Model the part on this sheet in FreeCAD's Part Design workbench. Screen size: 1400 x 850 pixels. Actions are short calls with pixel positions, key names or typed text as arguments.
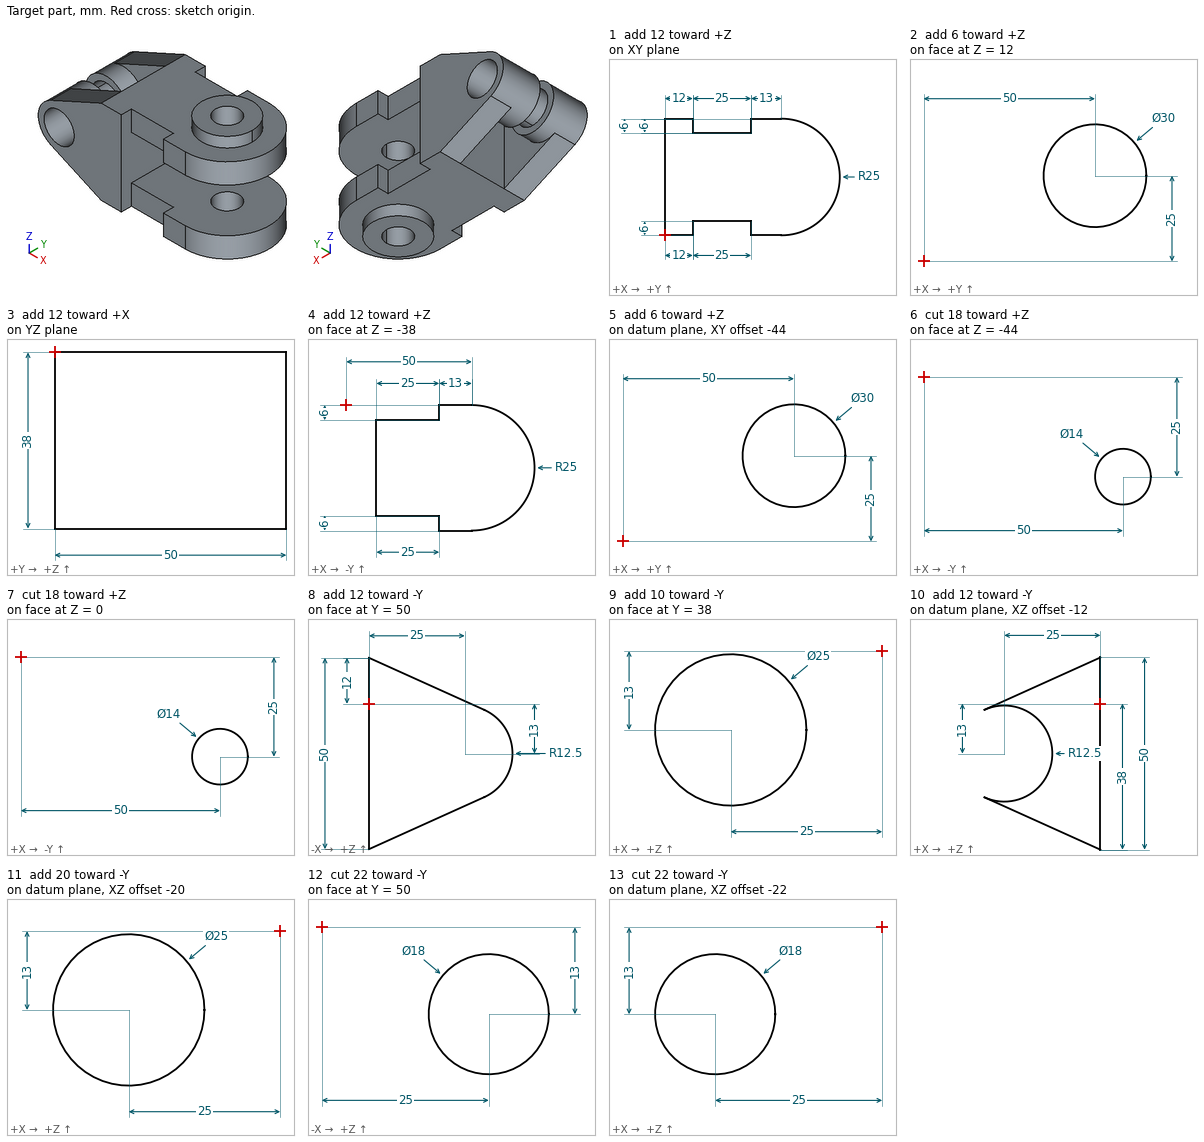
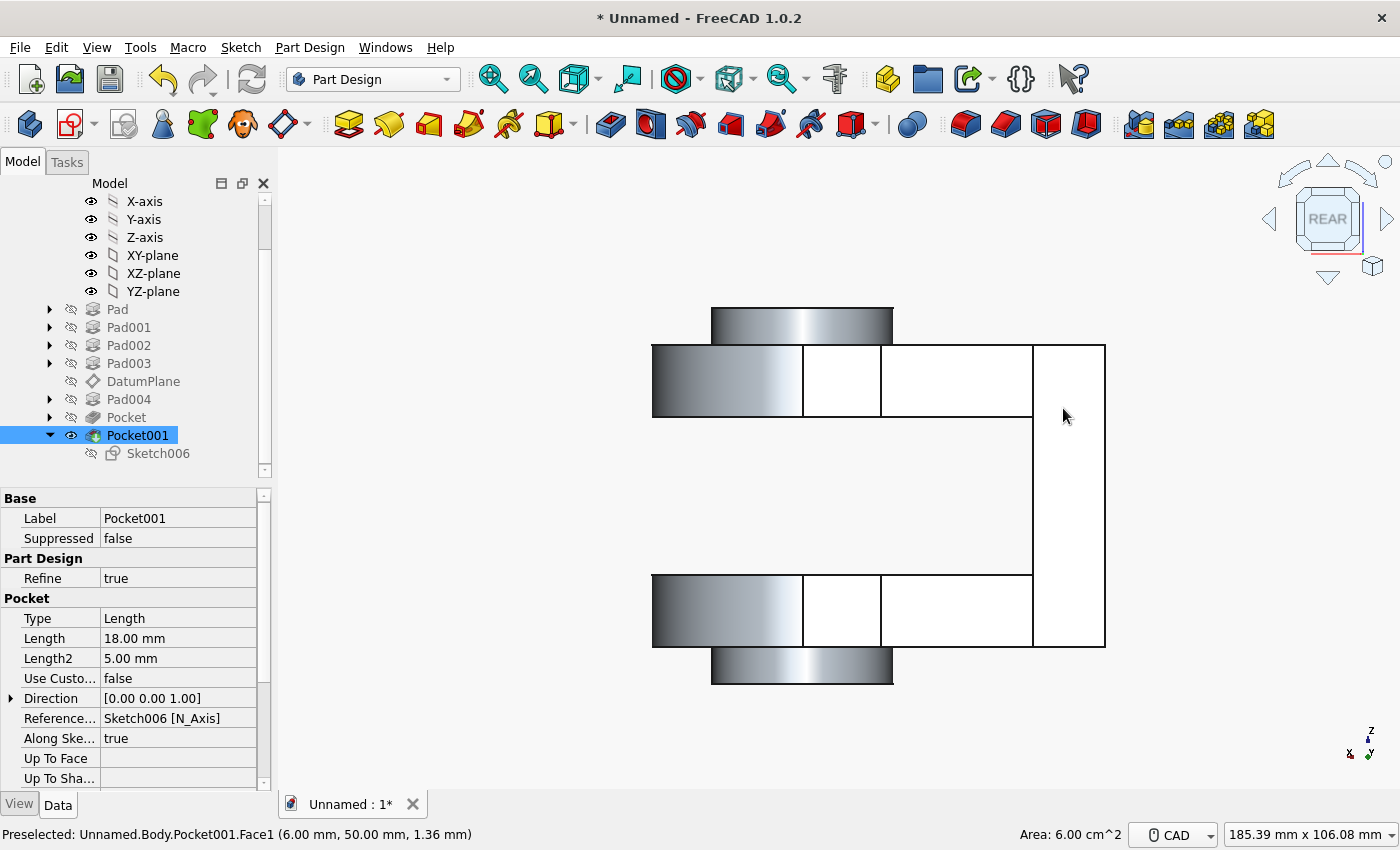
click(70, 124)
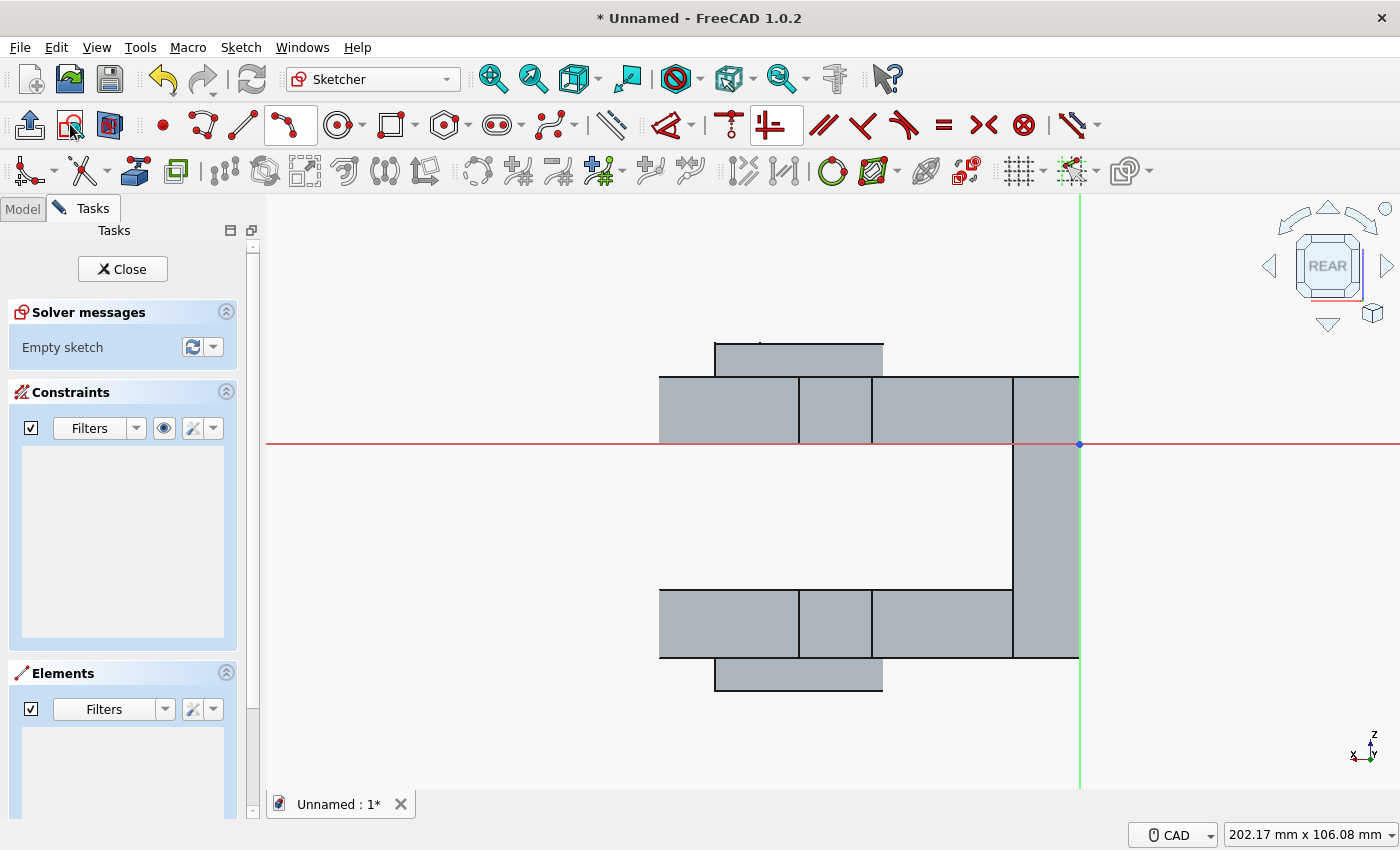
scroll(294, 375, down, 1)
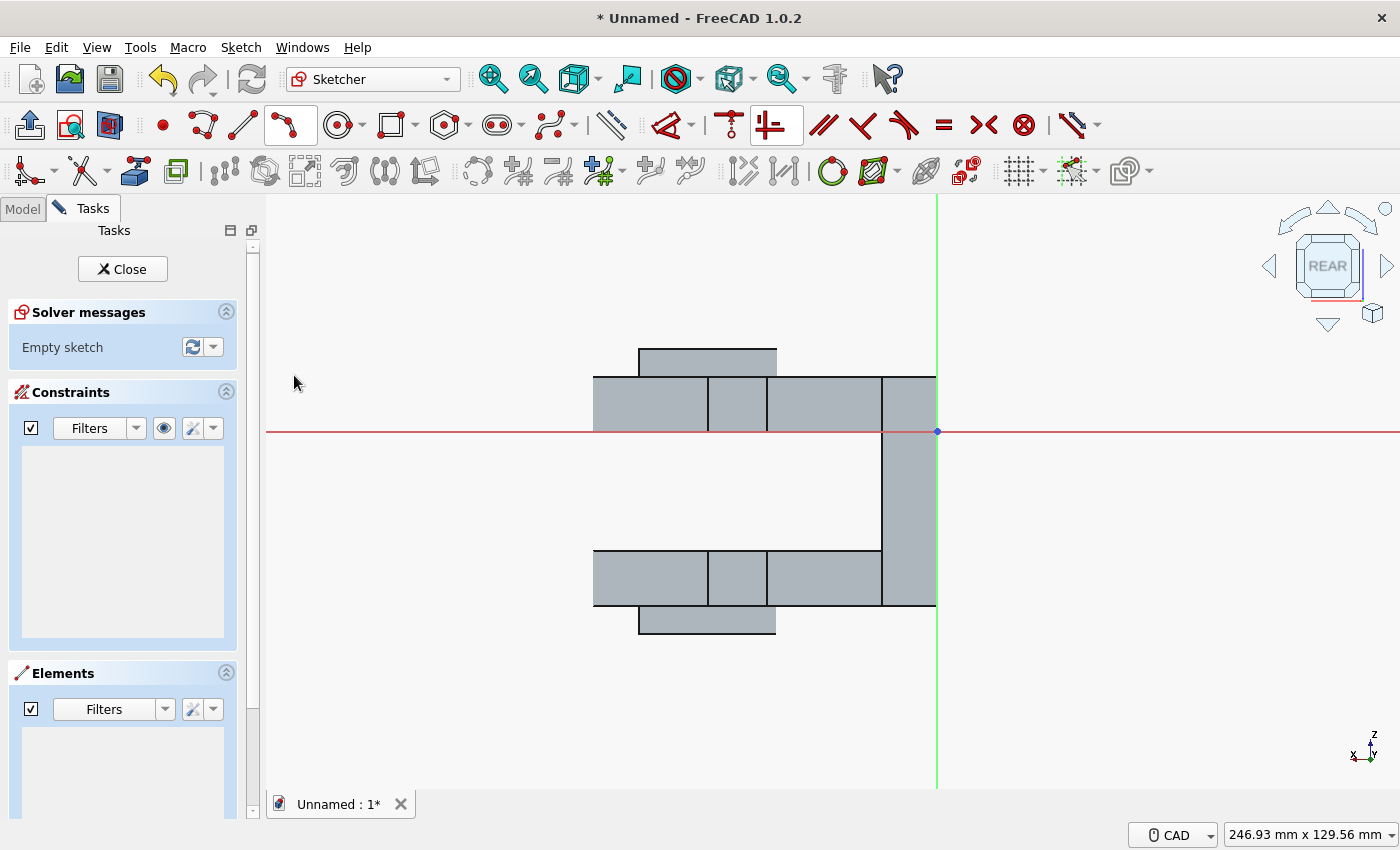
scroll(1235, 492, up, 3)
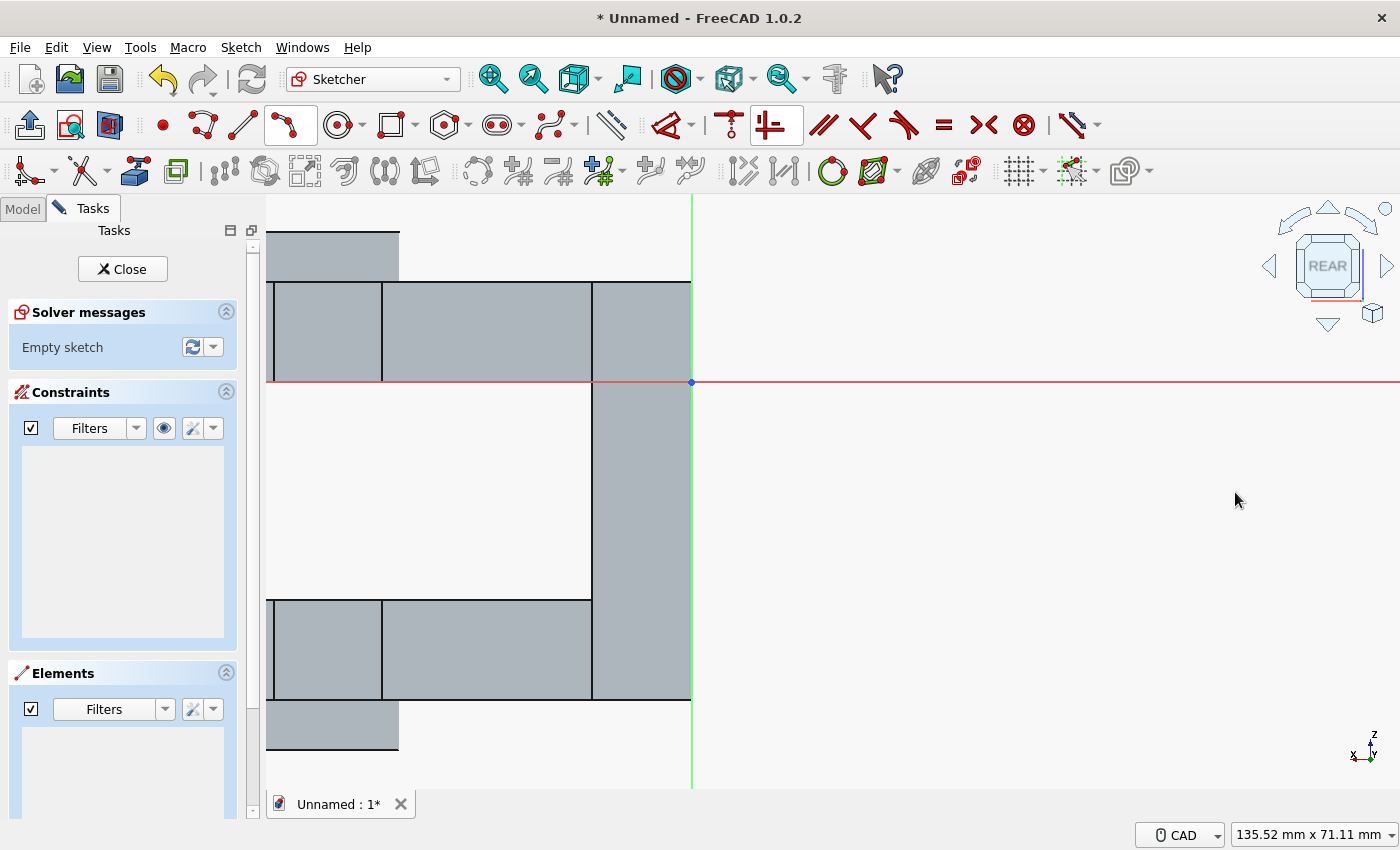
click(204, 126)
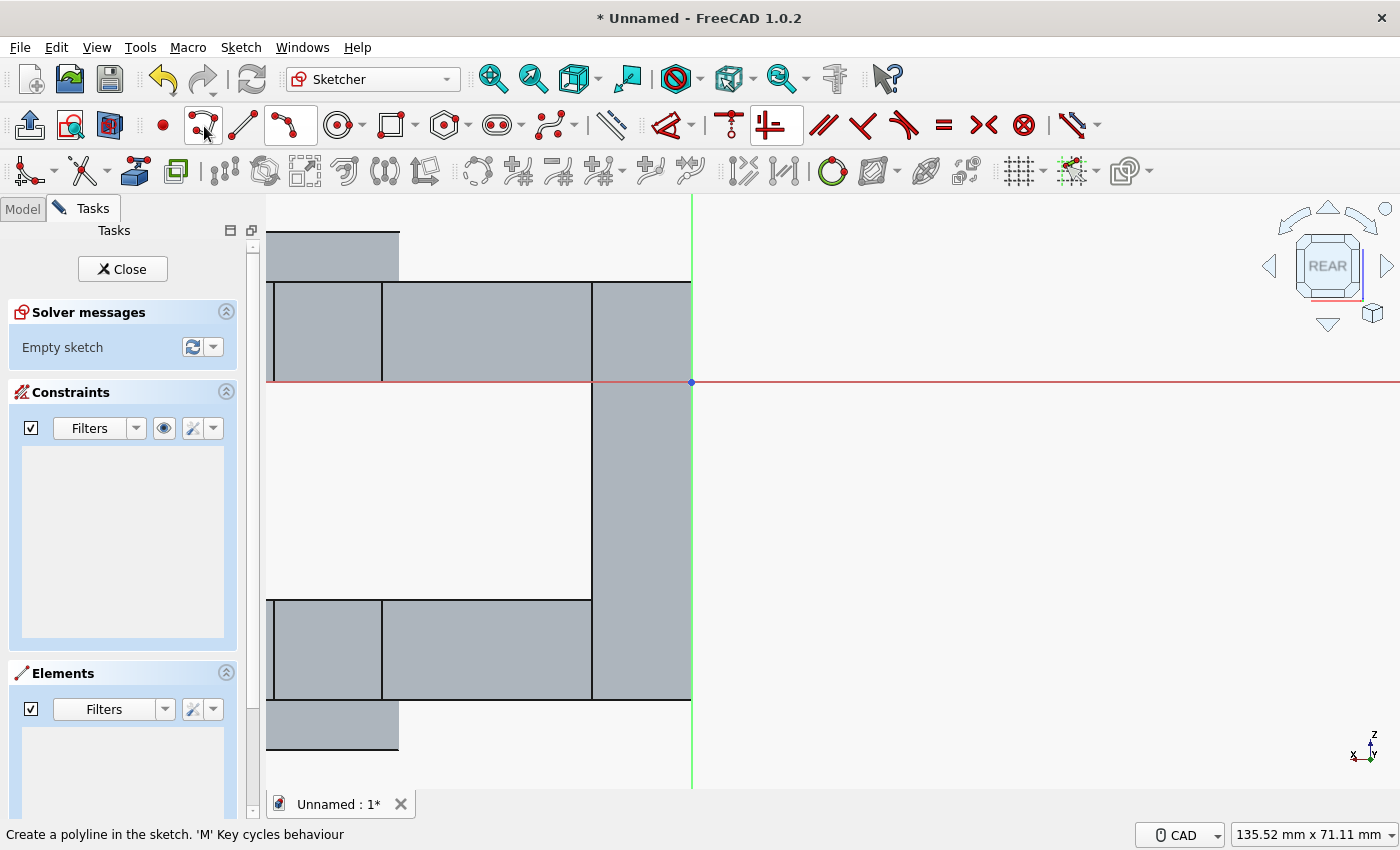
click(944, 396)
click(692, 282)
click(701, 700)
click(944, 586)
right_click(944, 586)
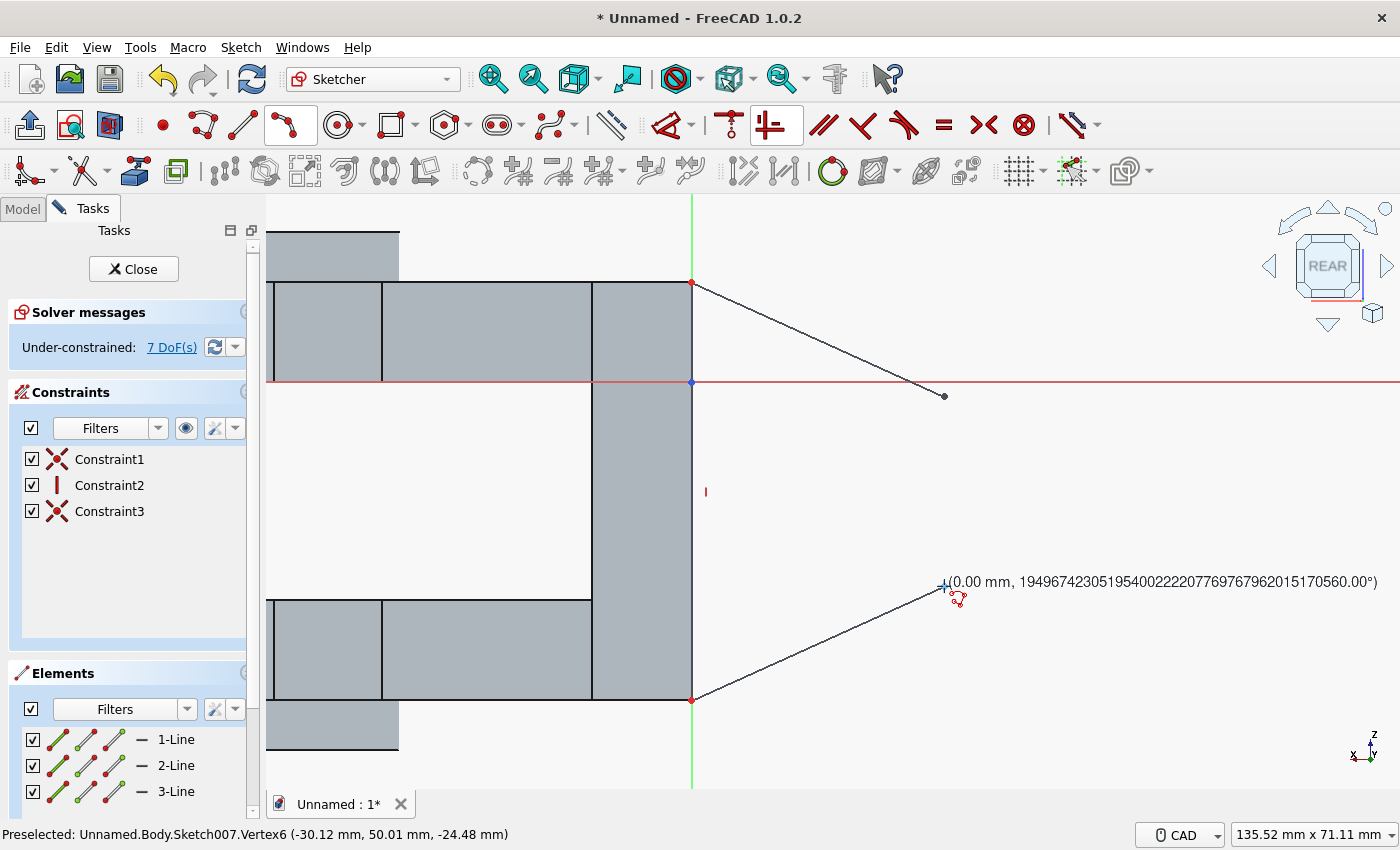
click(284, 126)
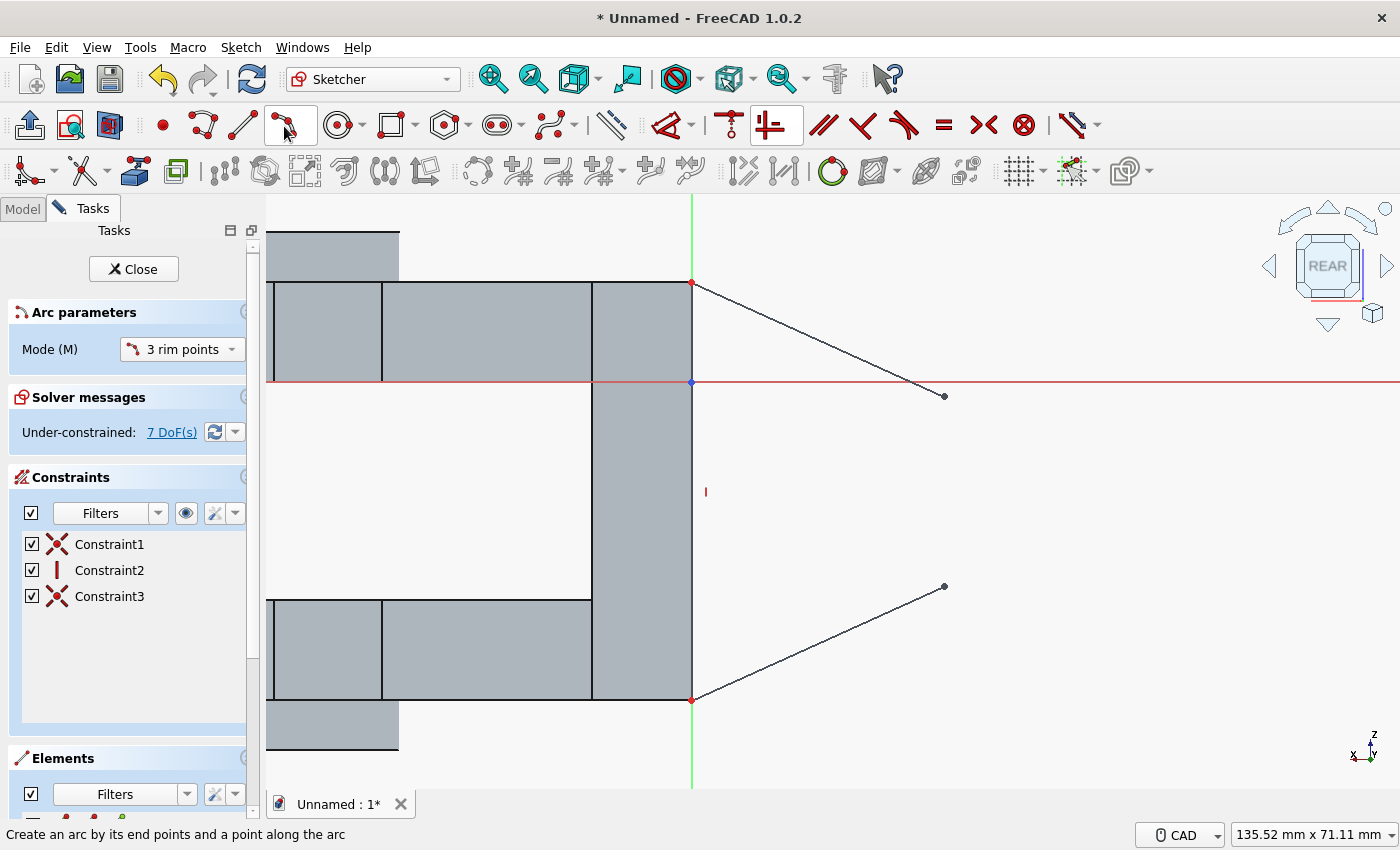
click(944, 587)
click(944, 397)
click(1006, 491)
key(Escape)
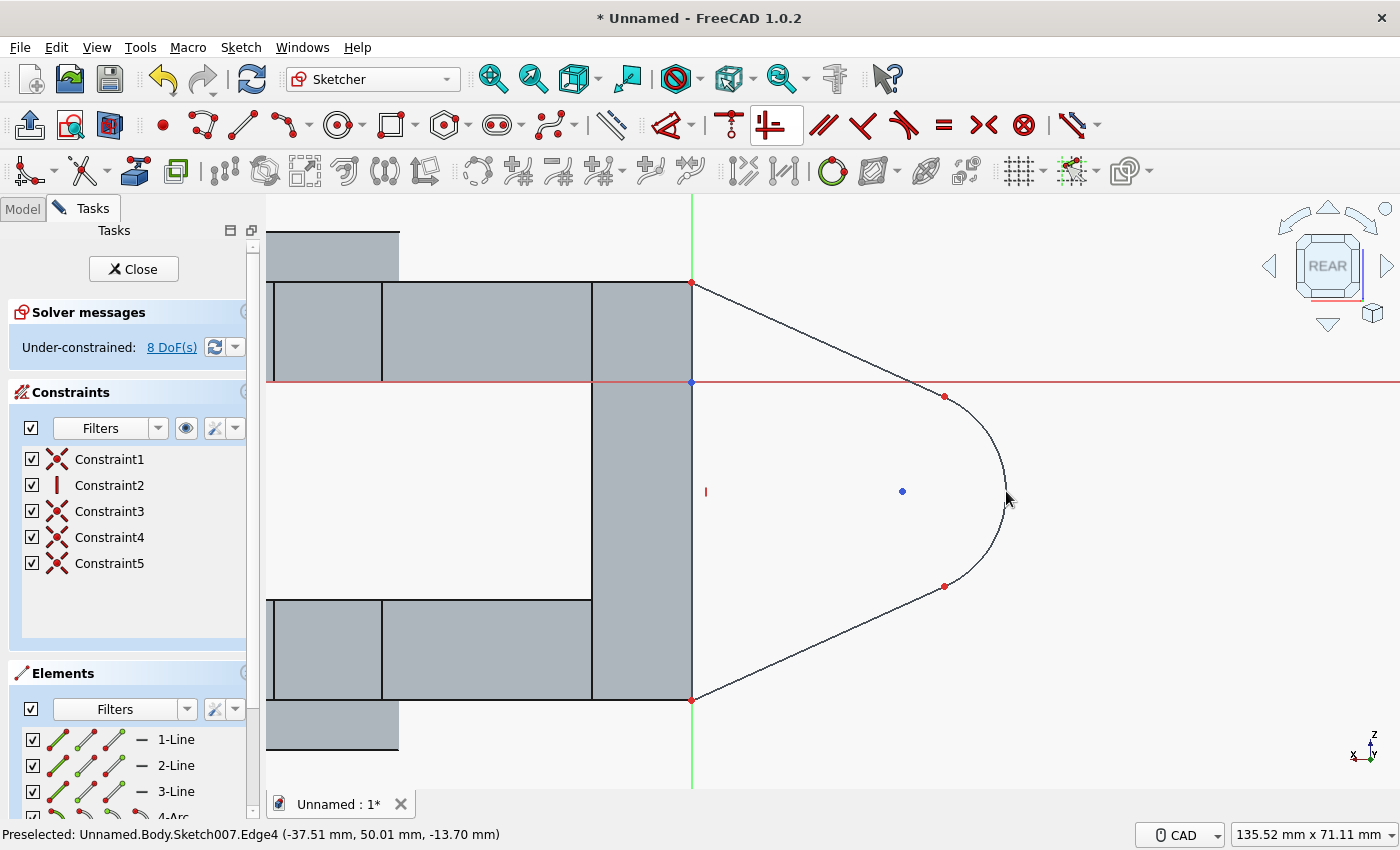
click(868, 363)